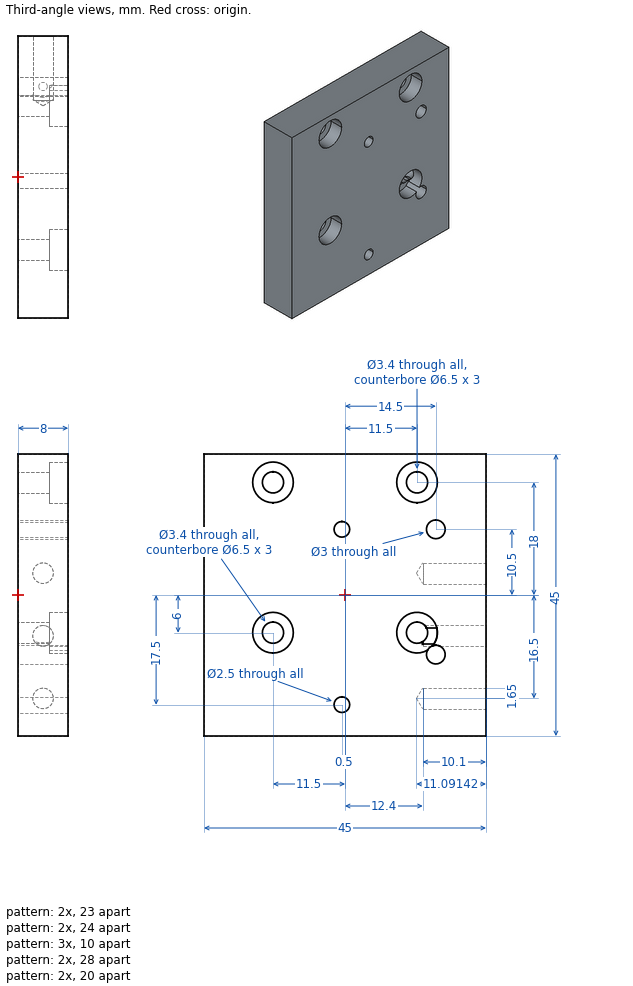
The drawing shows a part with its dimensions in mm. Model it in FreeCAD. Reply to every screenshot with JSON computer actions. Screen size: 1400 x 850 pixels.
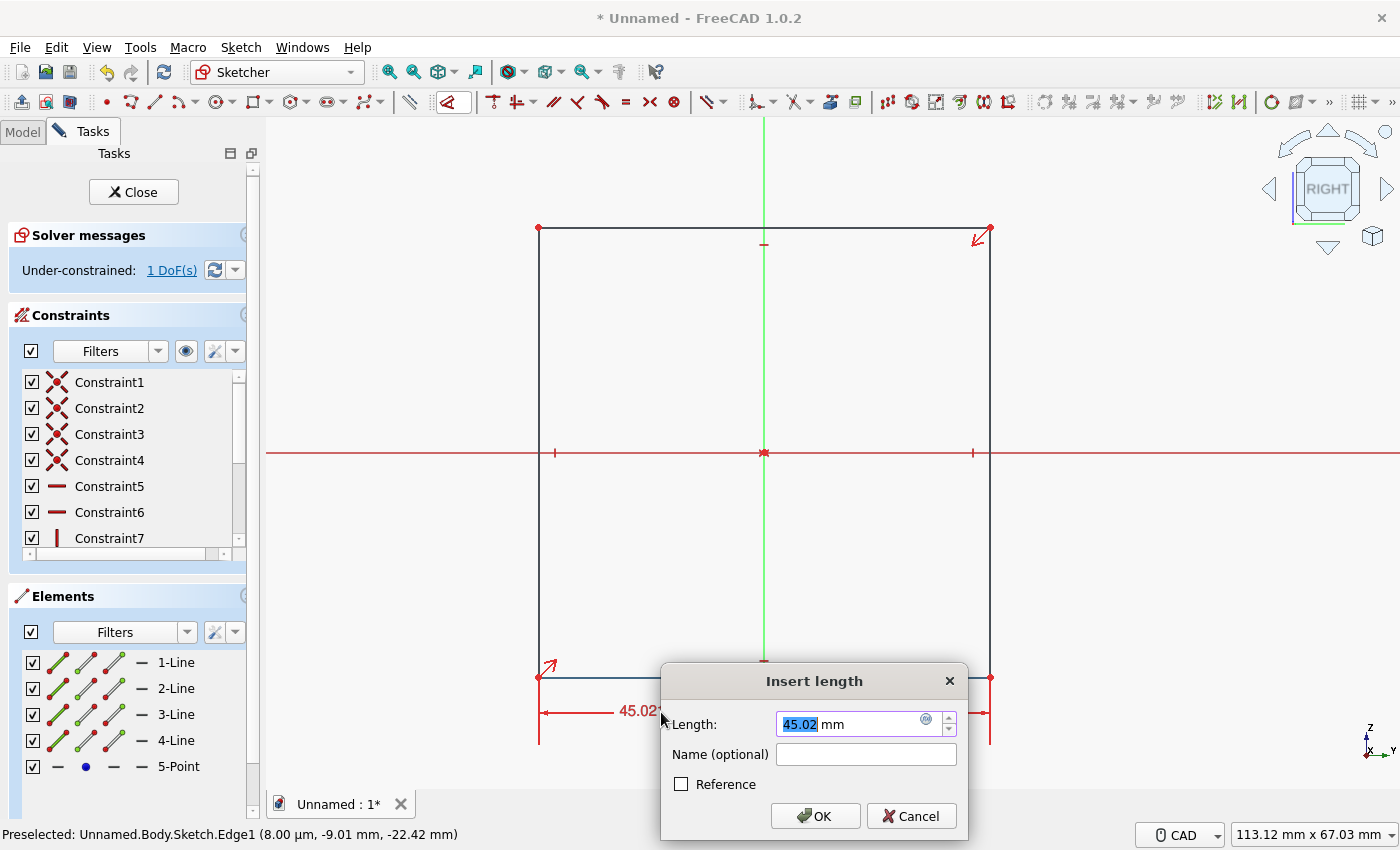
{"action": "type", "text": "45"}
{"action": "key", "text": "Return"}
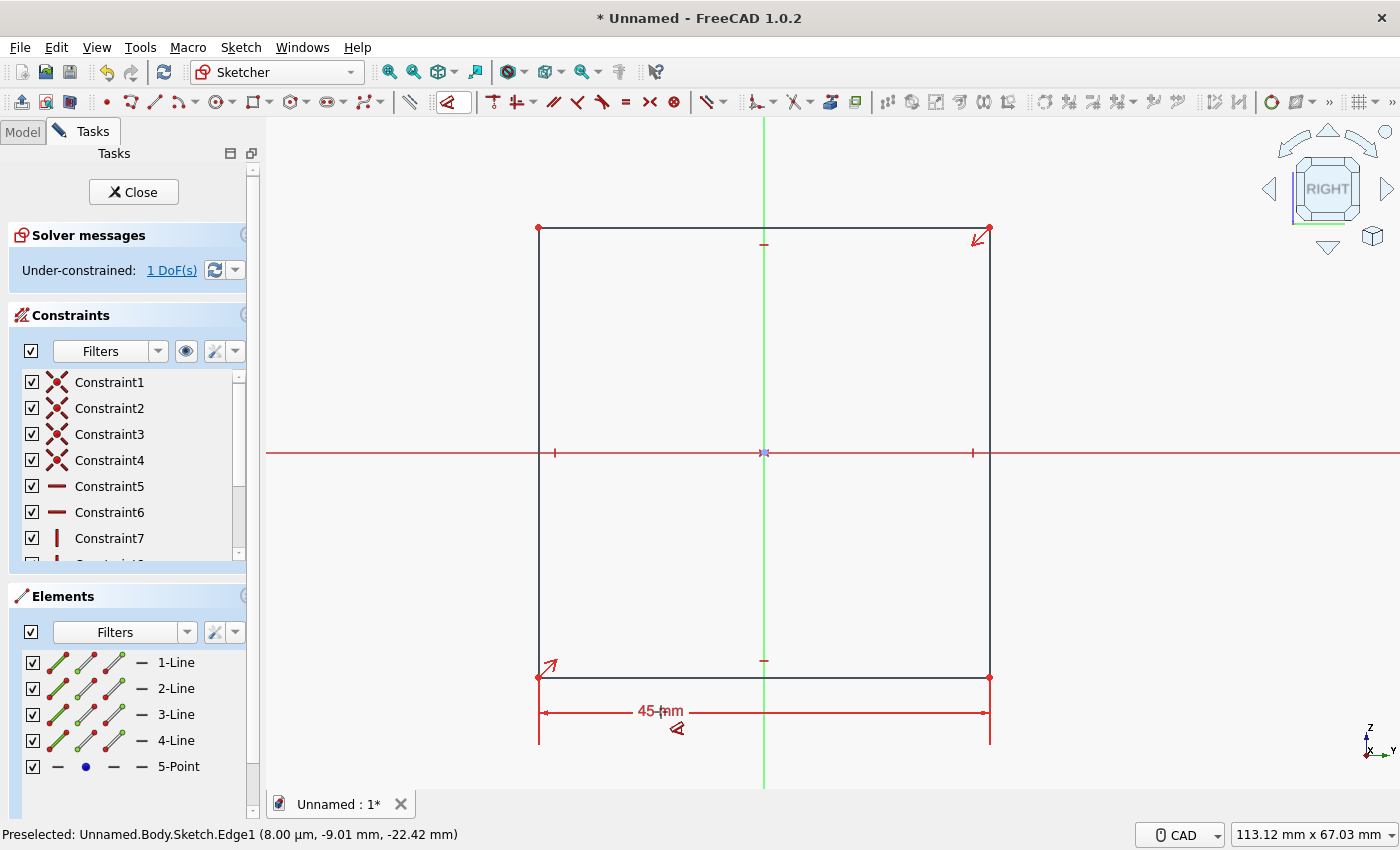
{"action": "left_click", "coordinate": [990, 543]}
{"action": "left_click", "coordinate": [1024, 349]}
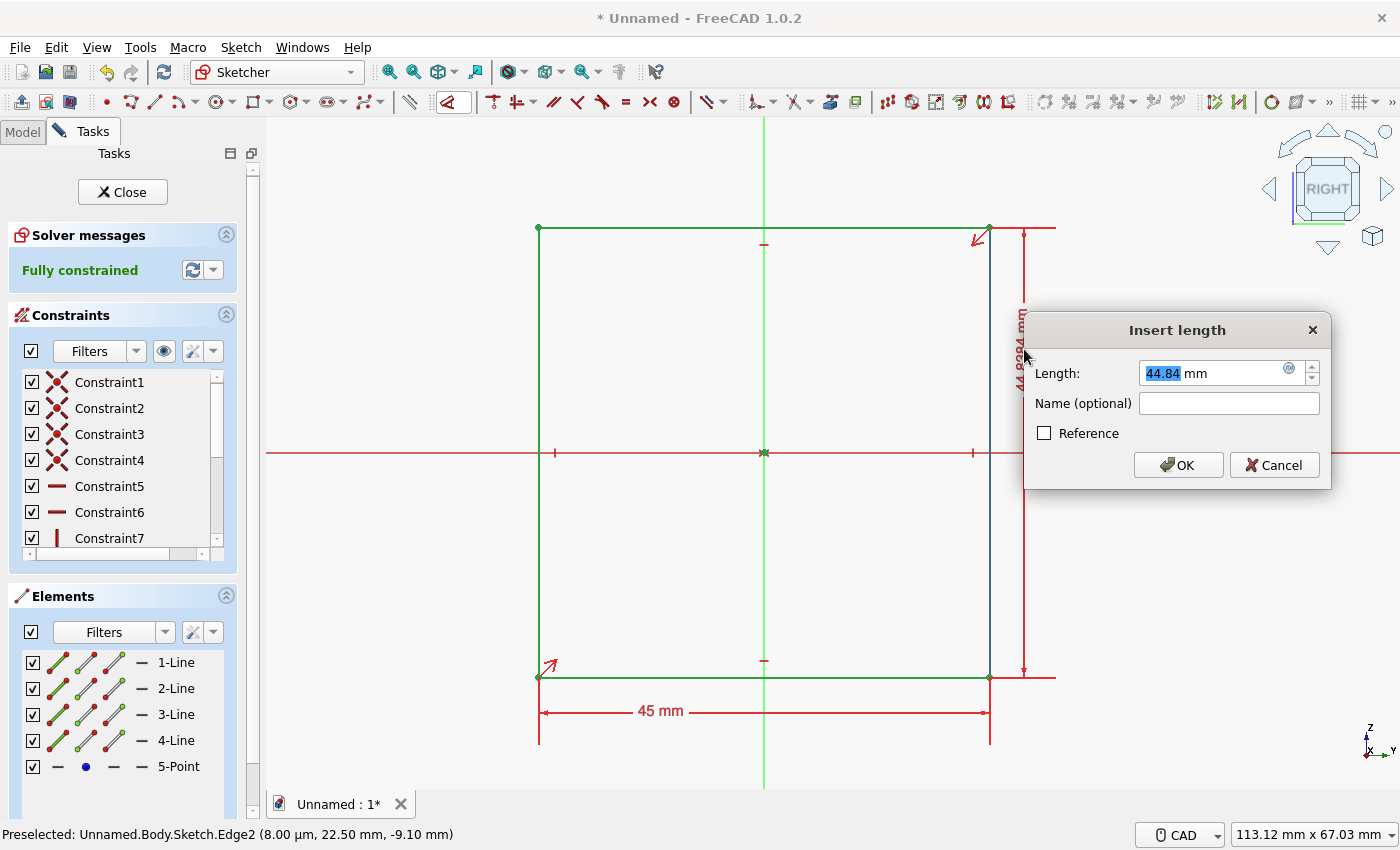
{"action": "type", "text": "45"}
{"action": "key", "text": "Return"}
{"action": "key", "text": "Escape"}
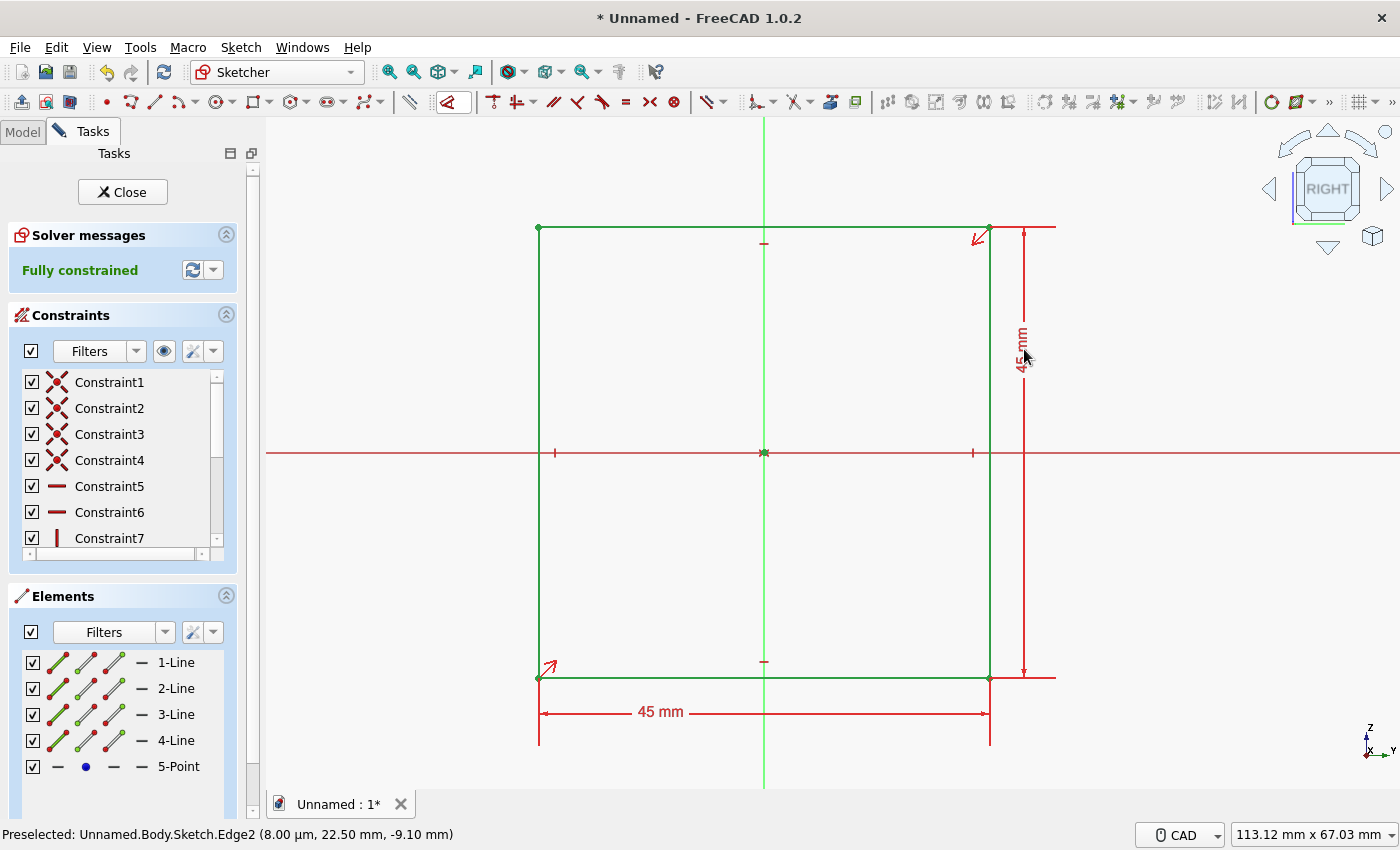
{"action": "left_click", "coordinate": [123, 192]}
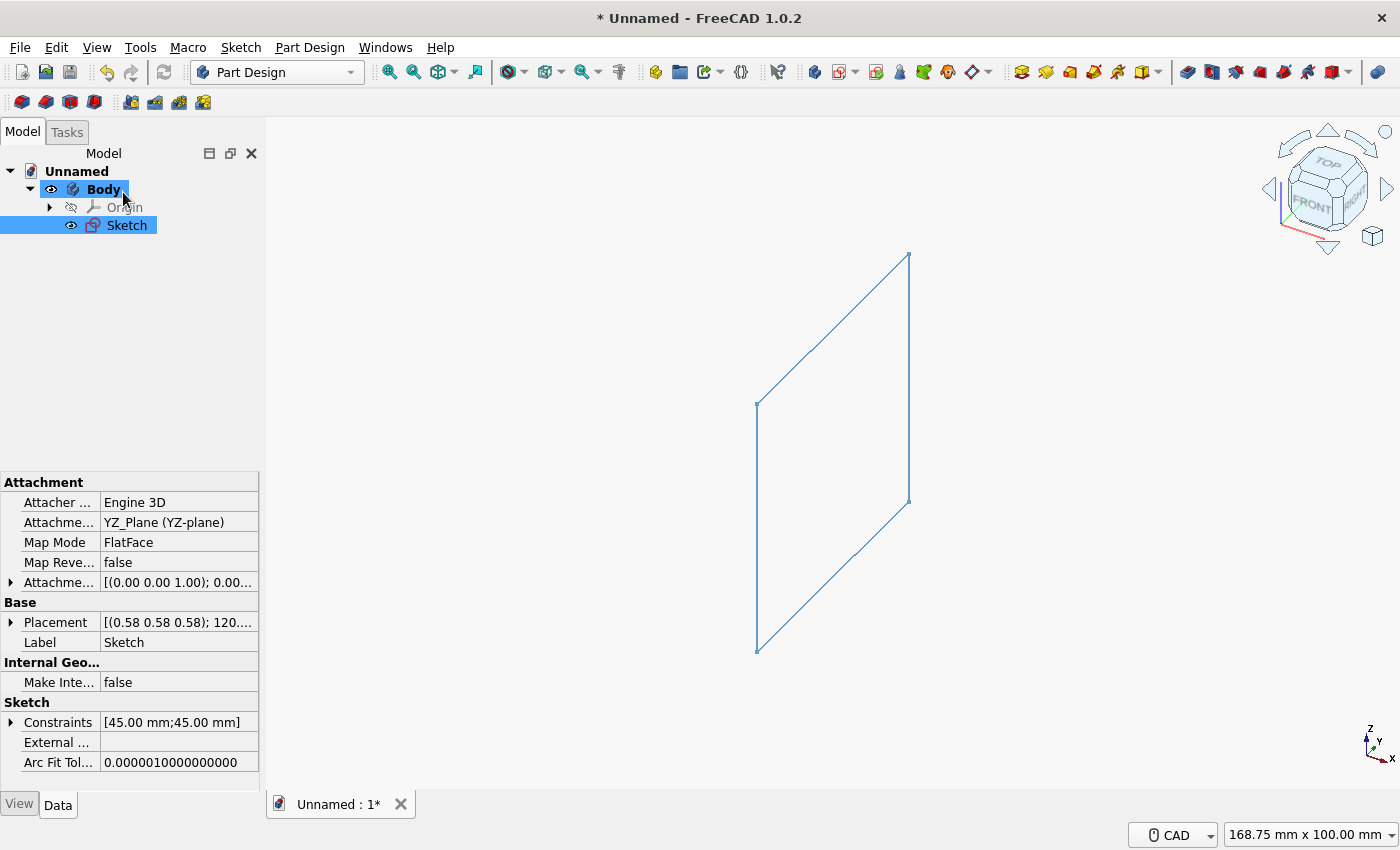
{"action": "left_click", "coordinate": [1022, 72]}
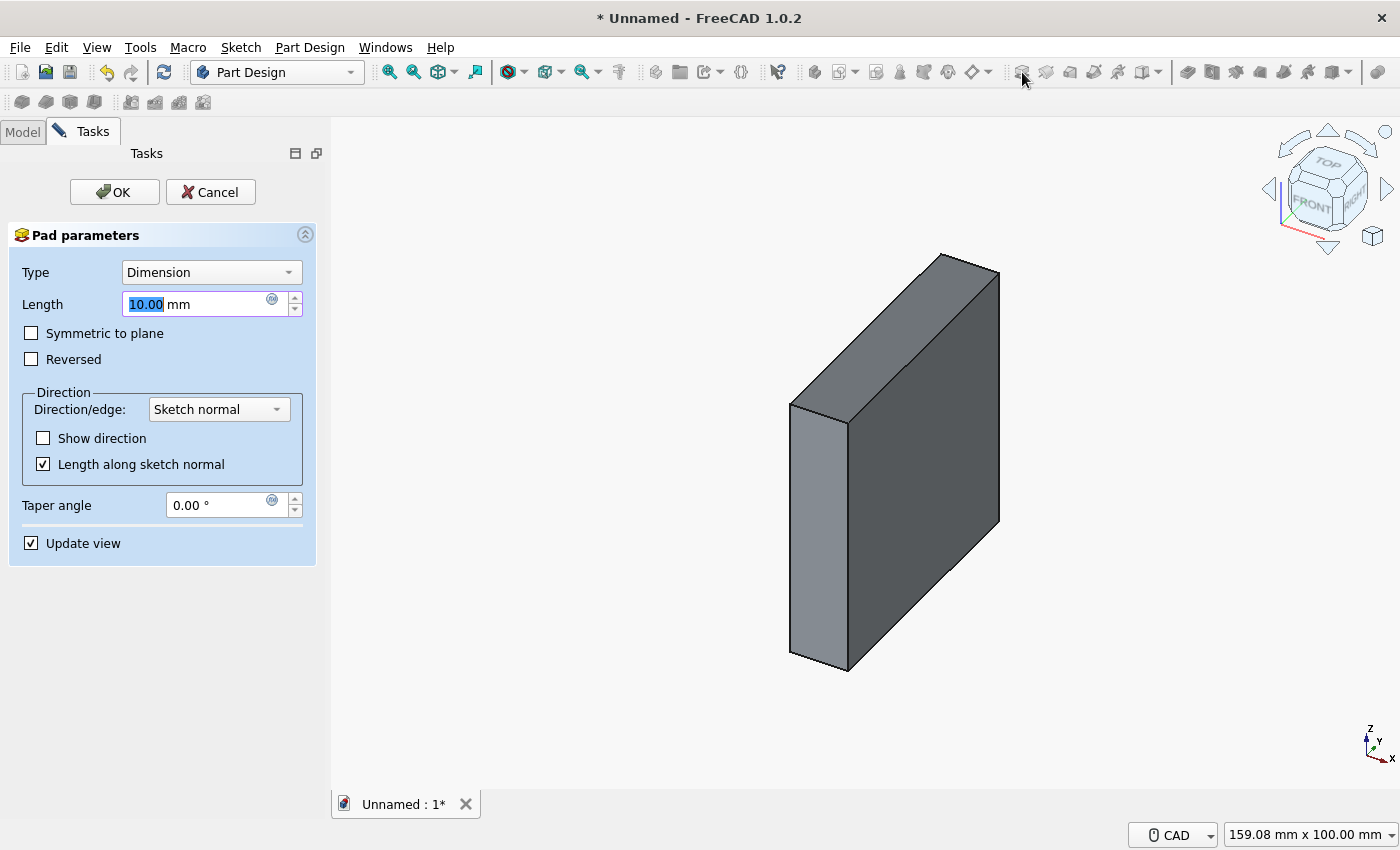
{"action": "type", "text": "8"}
{"action": "key", "text": "Tab"}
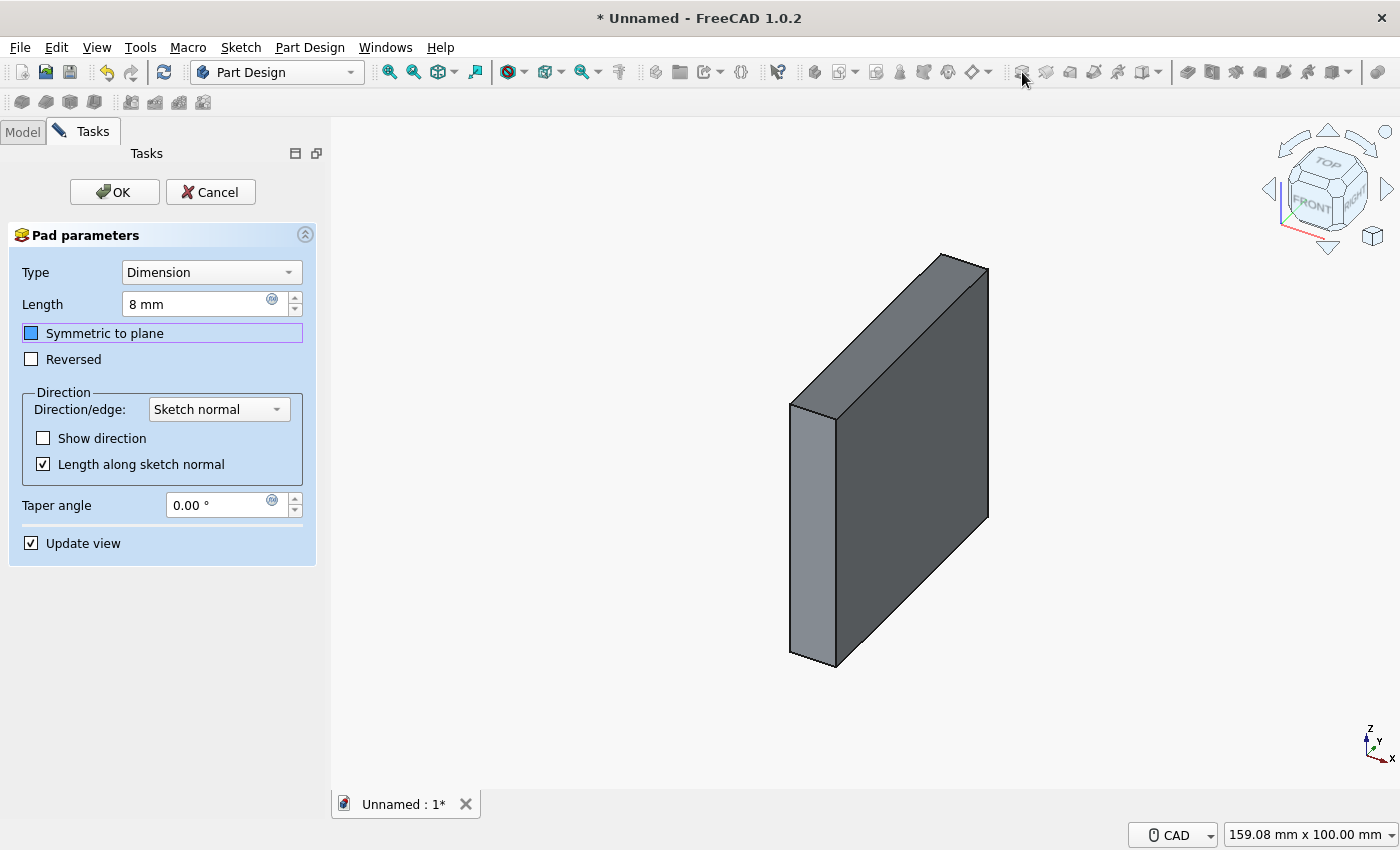
{"action": "left_click", "coordinate": [115, 192]}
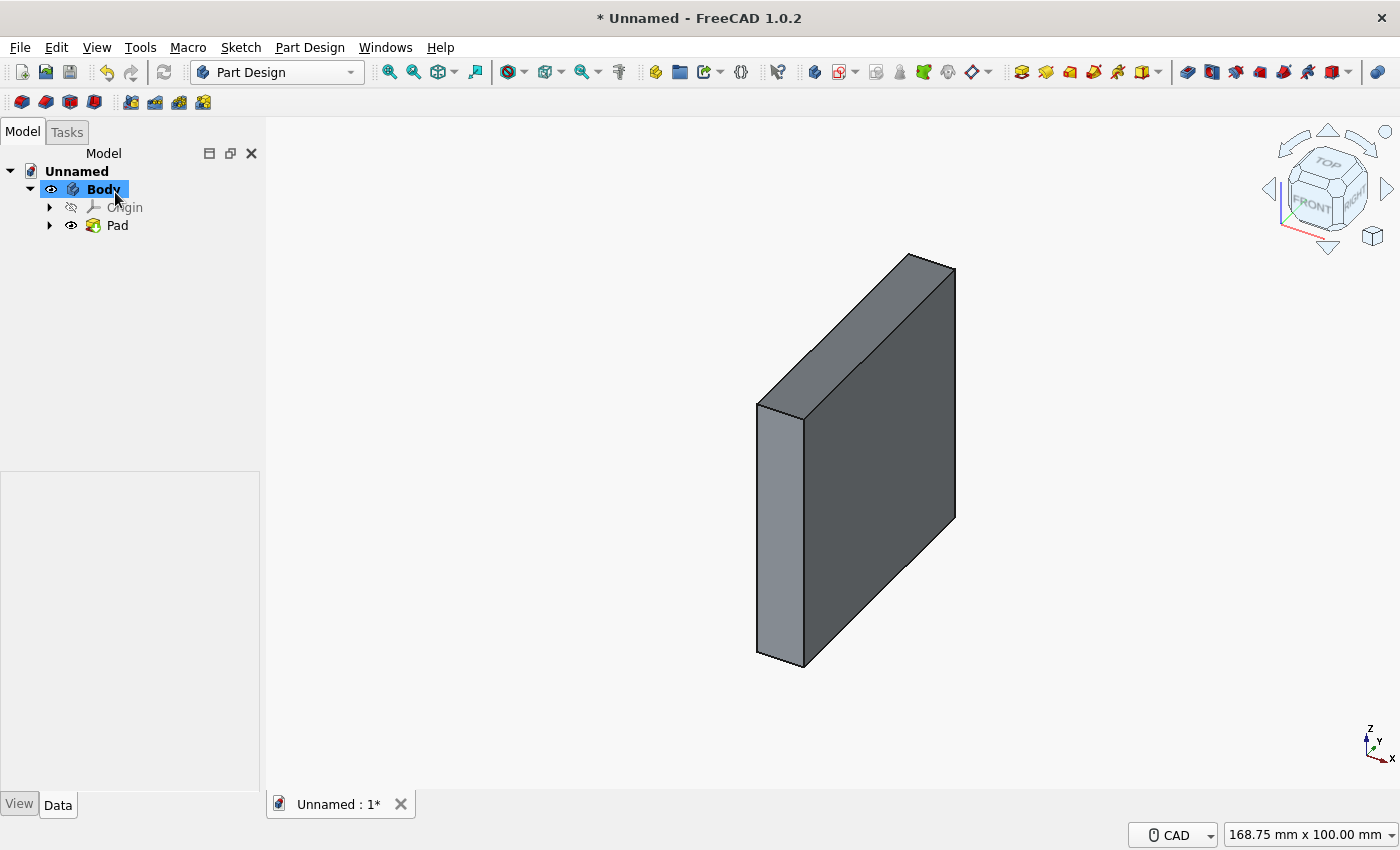
{"action": "left_click", "coordinate": [880, 467]}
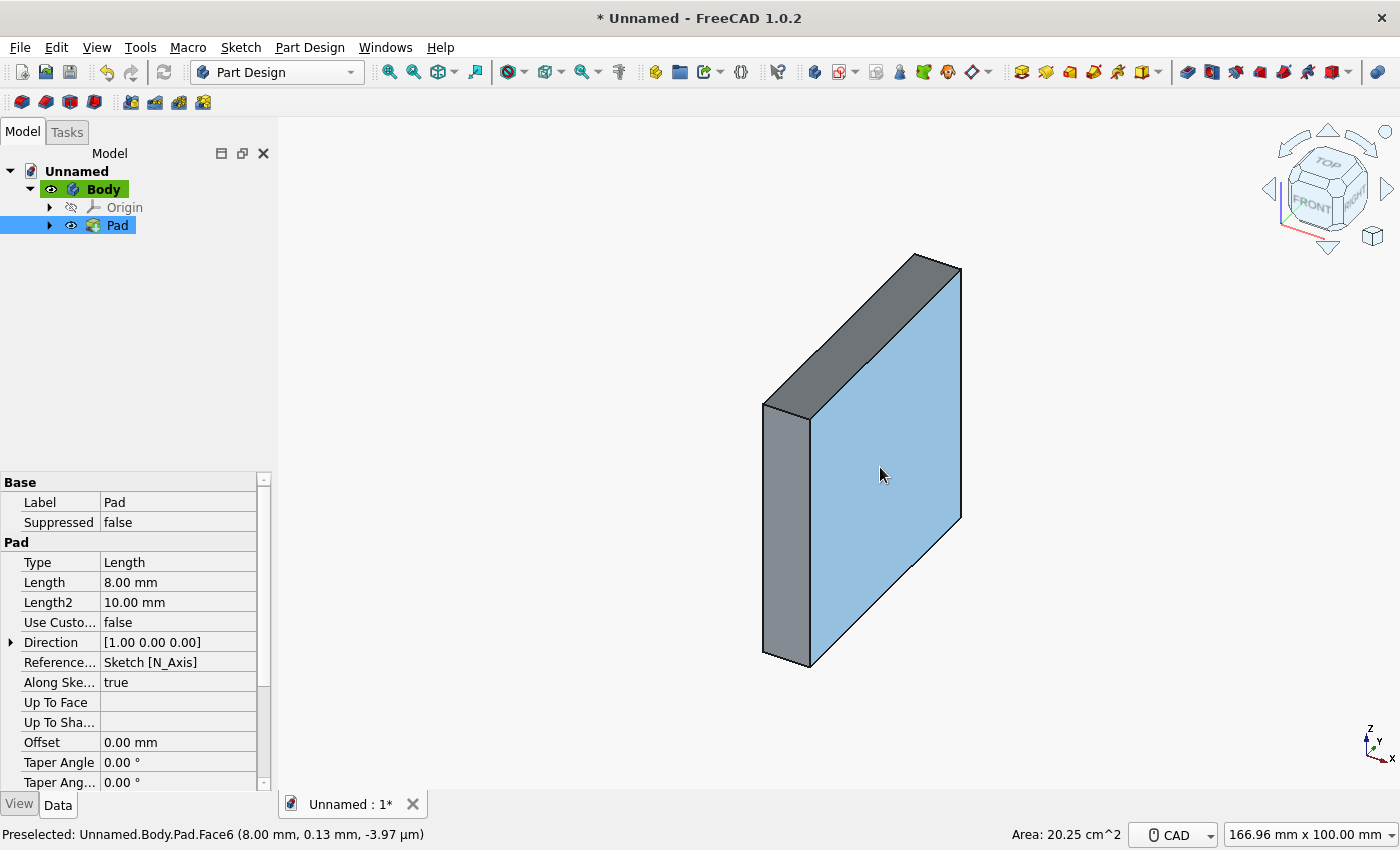
{"action": "left_click", "coordinate": [840, 72]}